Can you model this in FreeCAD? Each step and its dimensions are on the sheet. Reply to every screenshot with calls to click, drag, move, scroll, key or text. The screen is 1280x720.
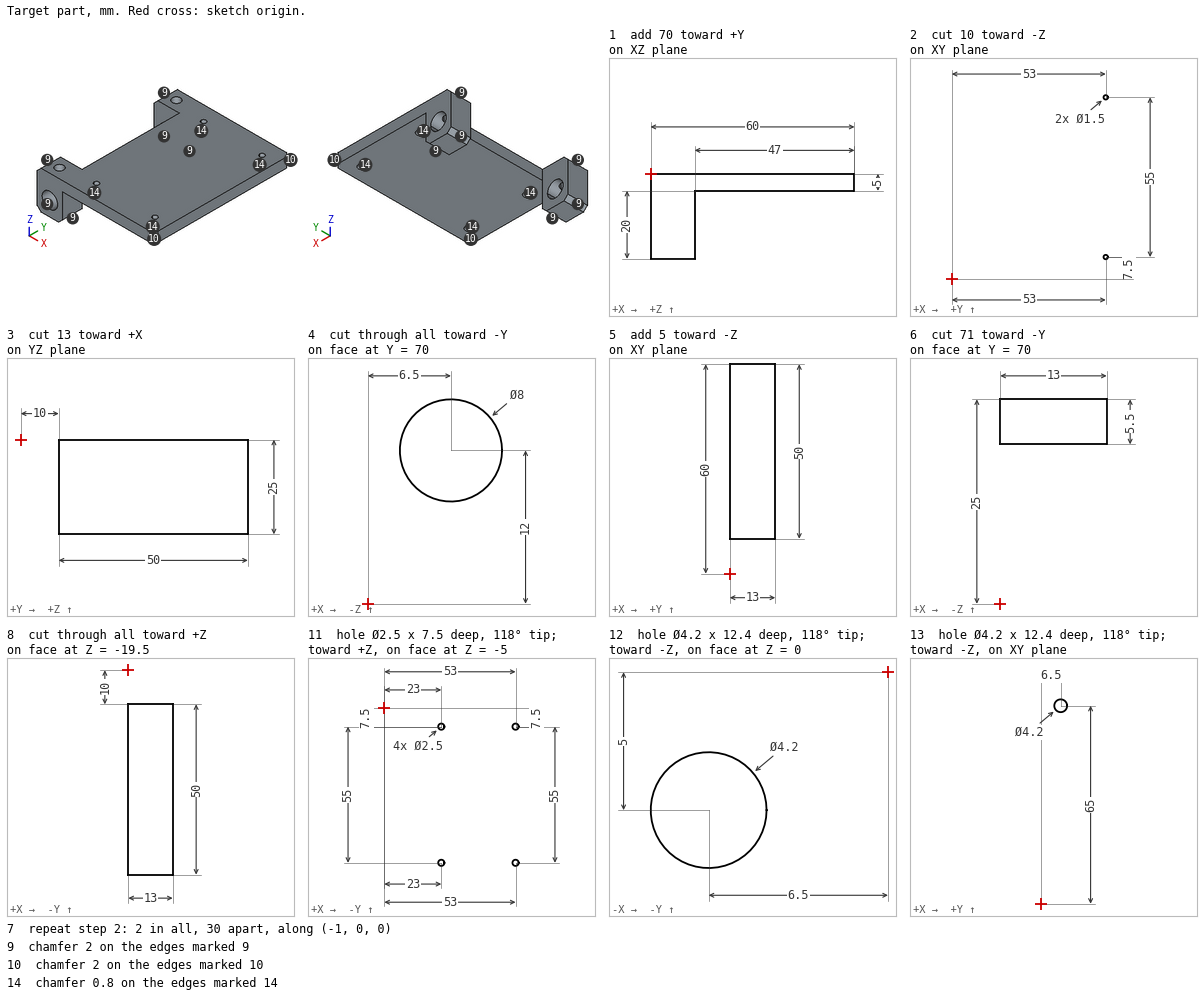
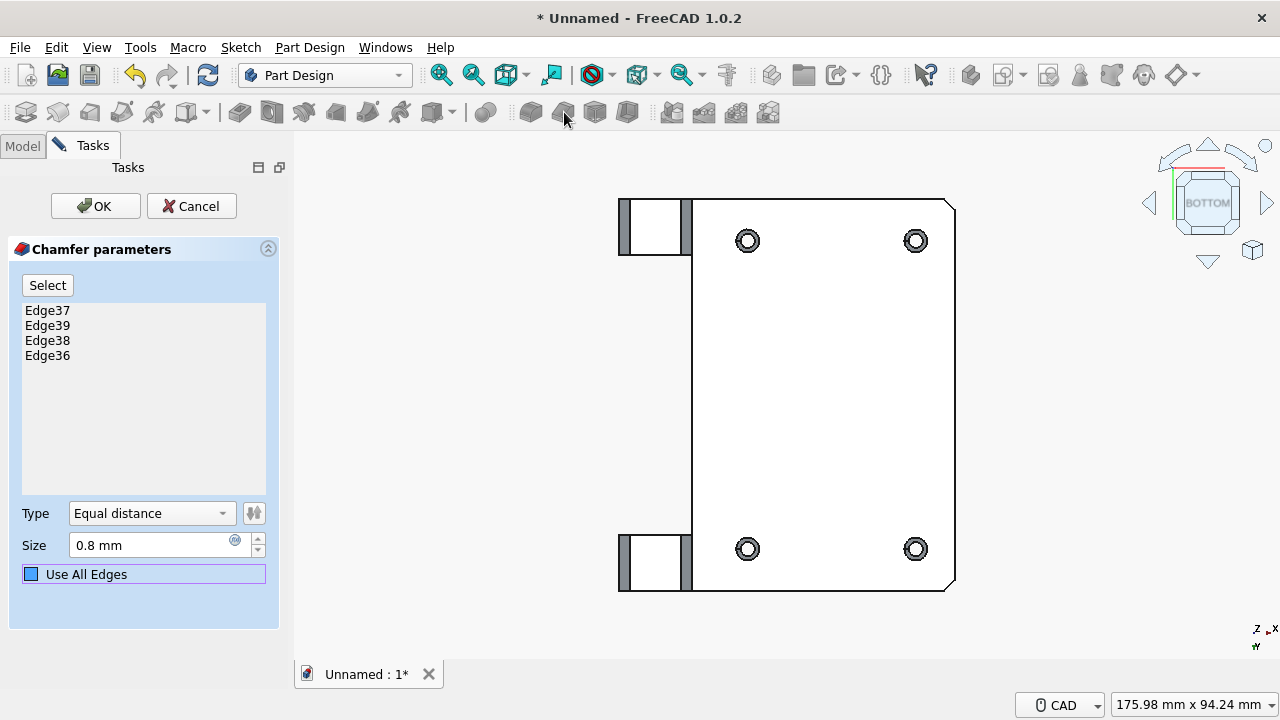
click(96, 206)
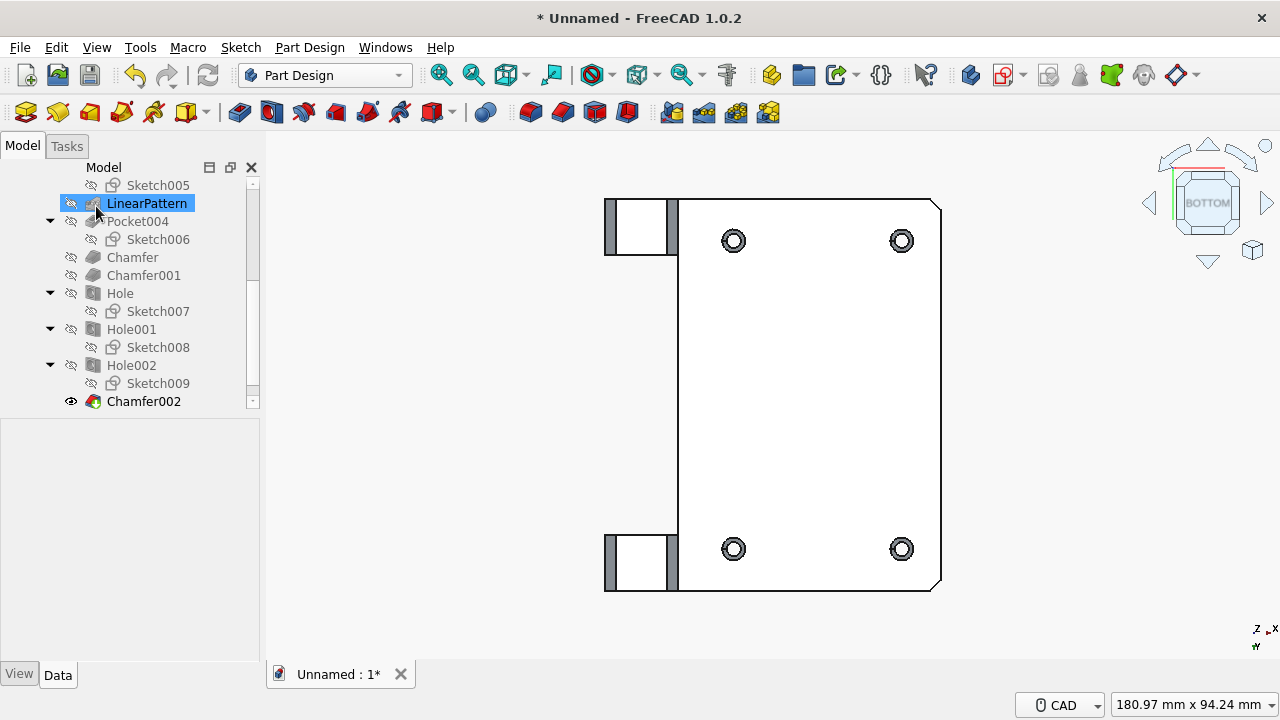
key(0)